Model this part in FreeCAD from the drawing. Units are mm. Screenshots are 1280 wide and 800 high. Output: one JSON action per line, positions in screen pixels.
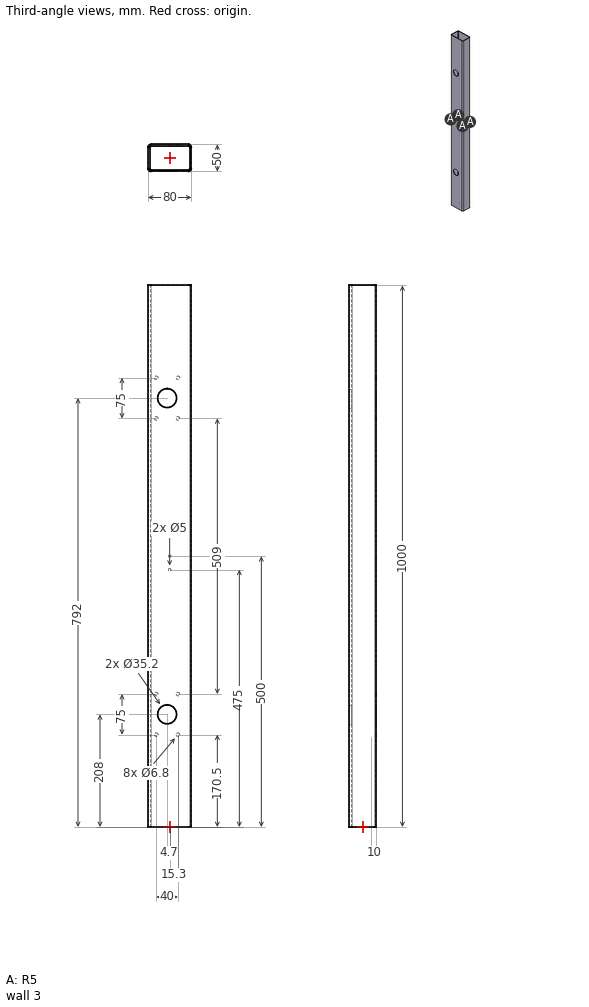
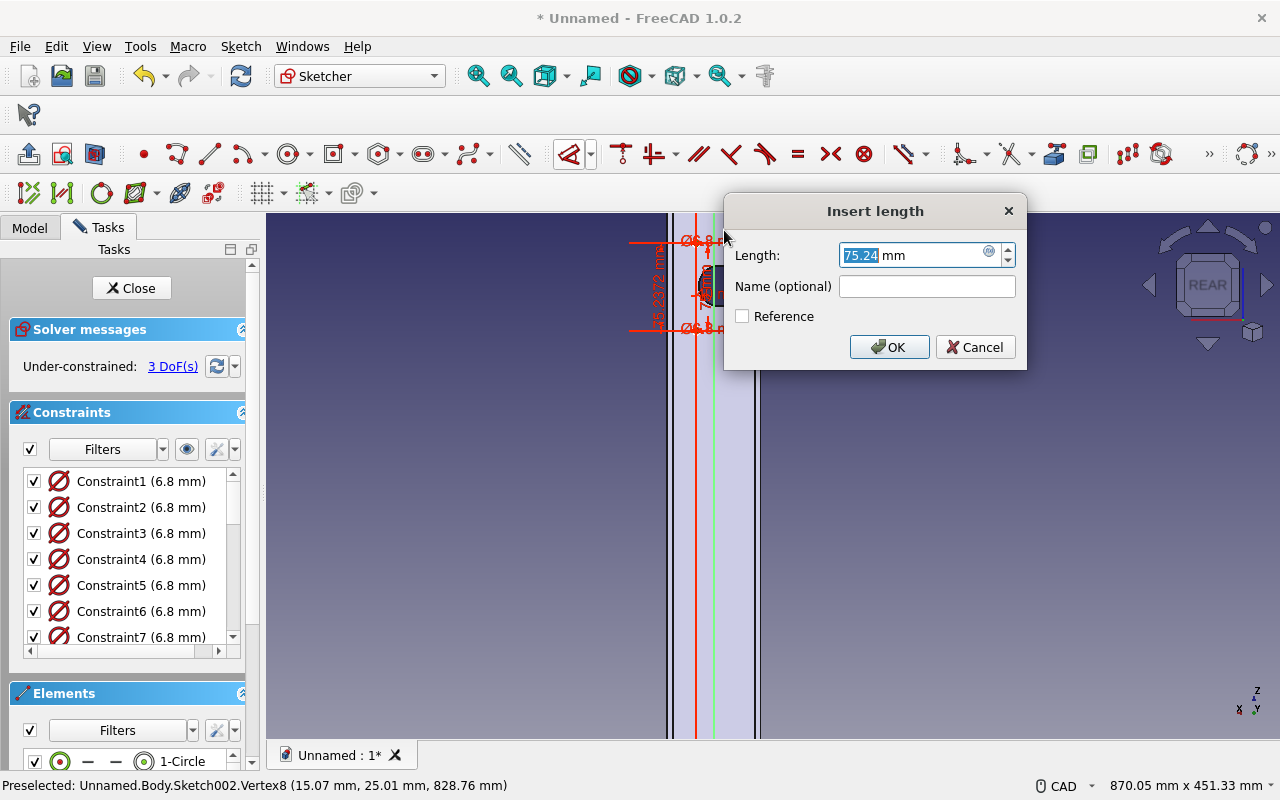
{"action": "type", "text": "75"}
{"action": "key", "text": "Return"}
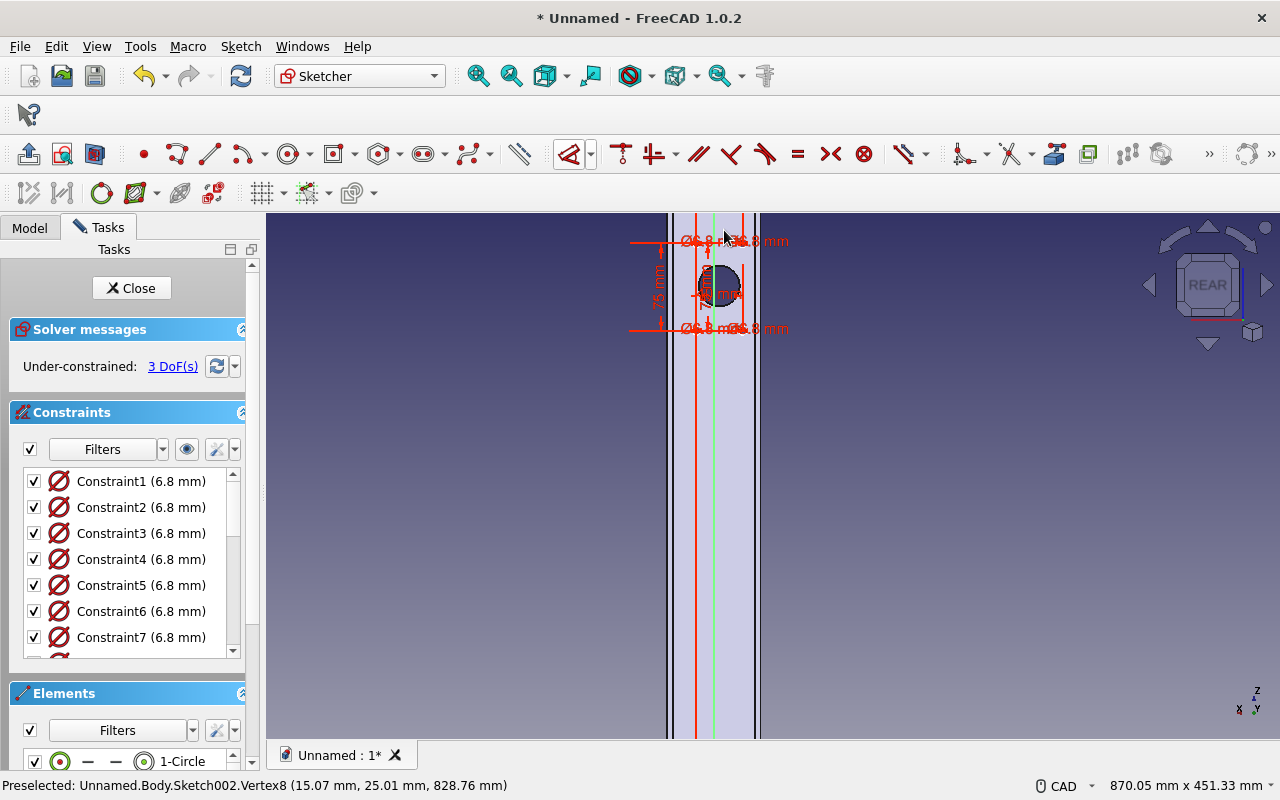
{"action": "scroll", "coordinate": [696, 332], "scroll_direction": "down", "scroll_amount": 5}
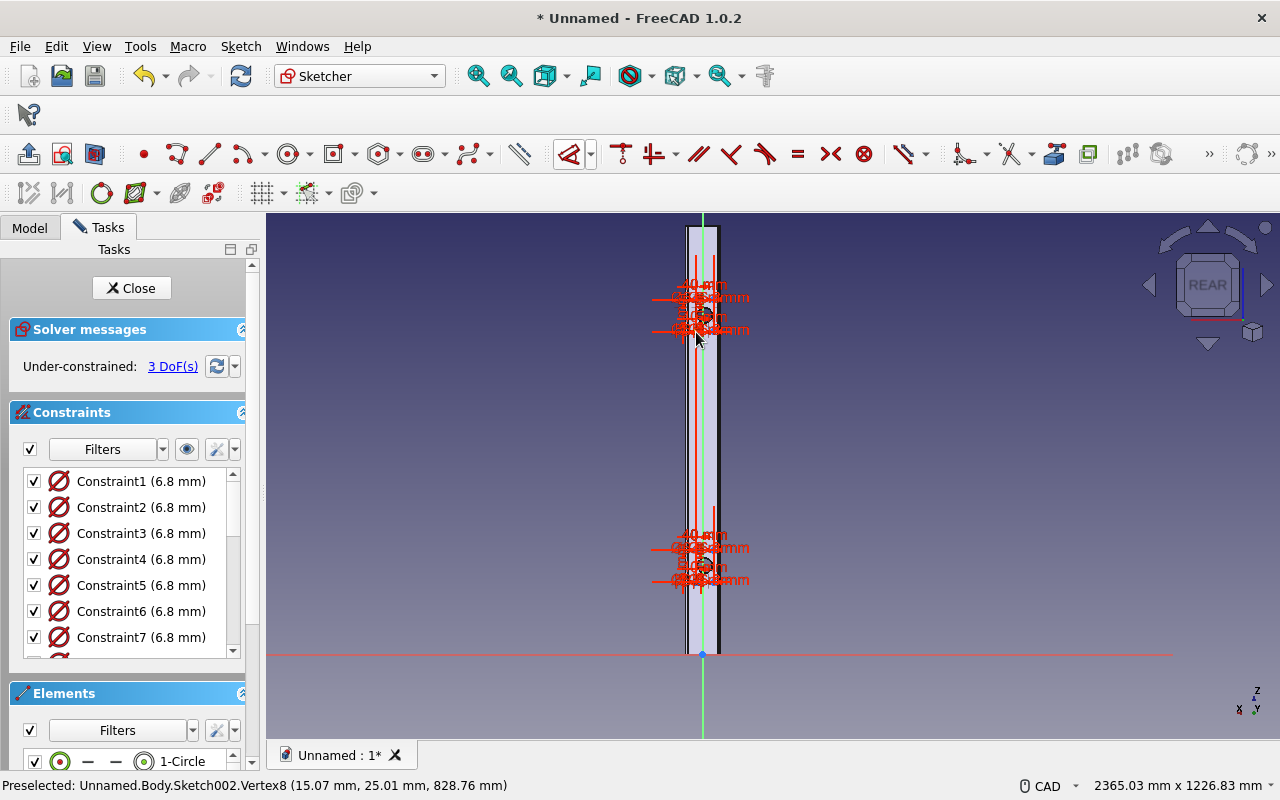
{"action": "scroll", "coordinate": [696, 582], "scroll_direction": "up", "scroll_amount": 10}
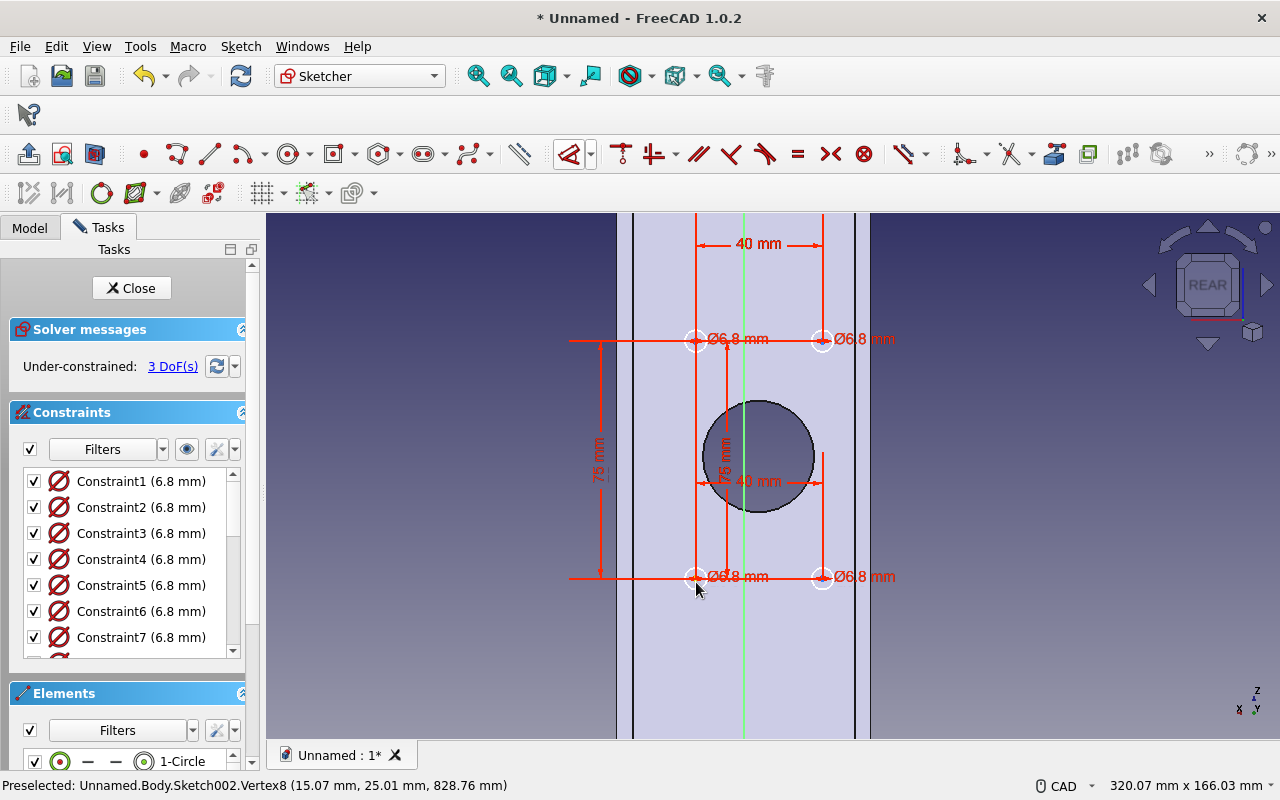
{"action": "left_click", "coordinate": [696, 579]}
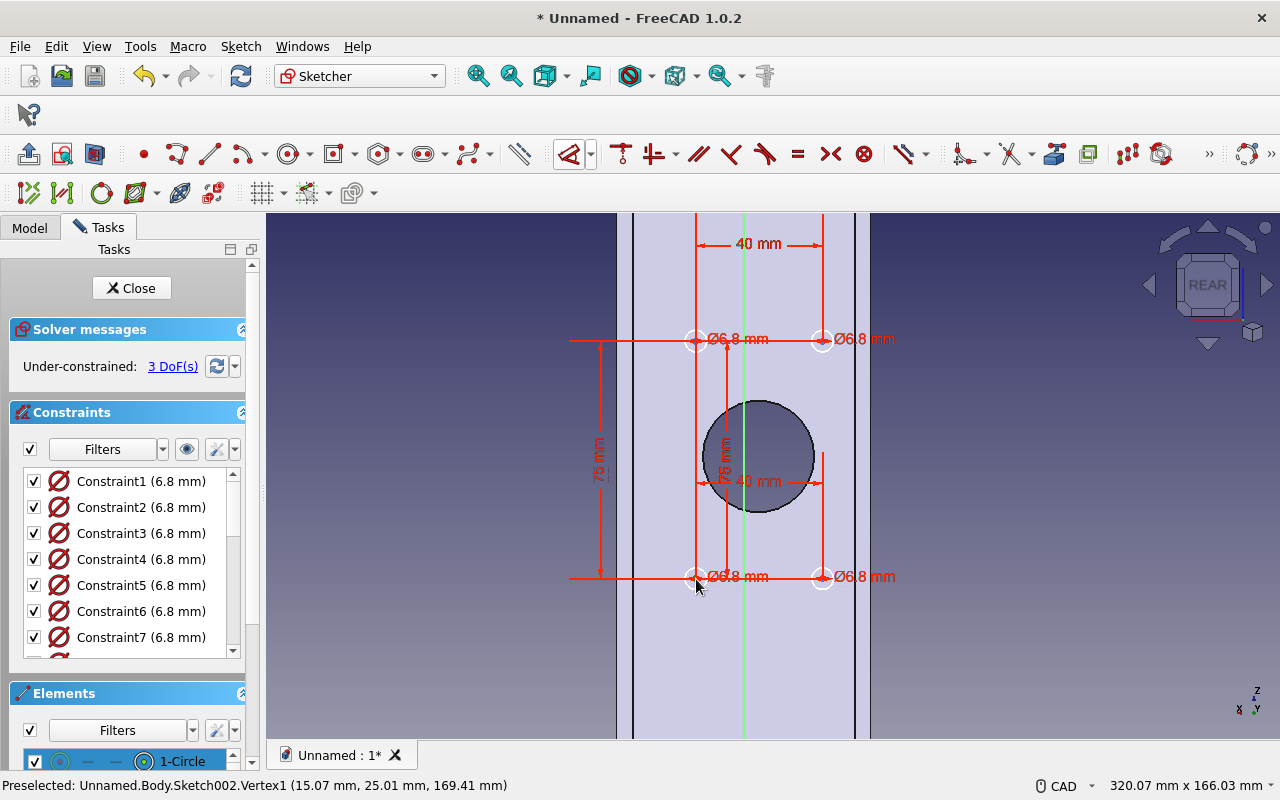
{"action": "left_click", "coordinate": [590, 154]}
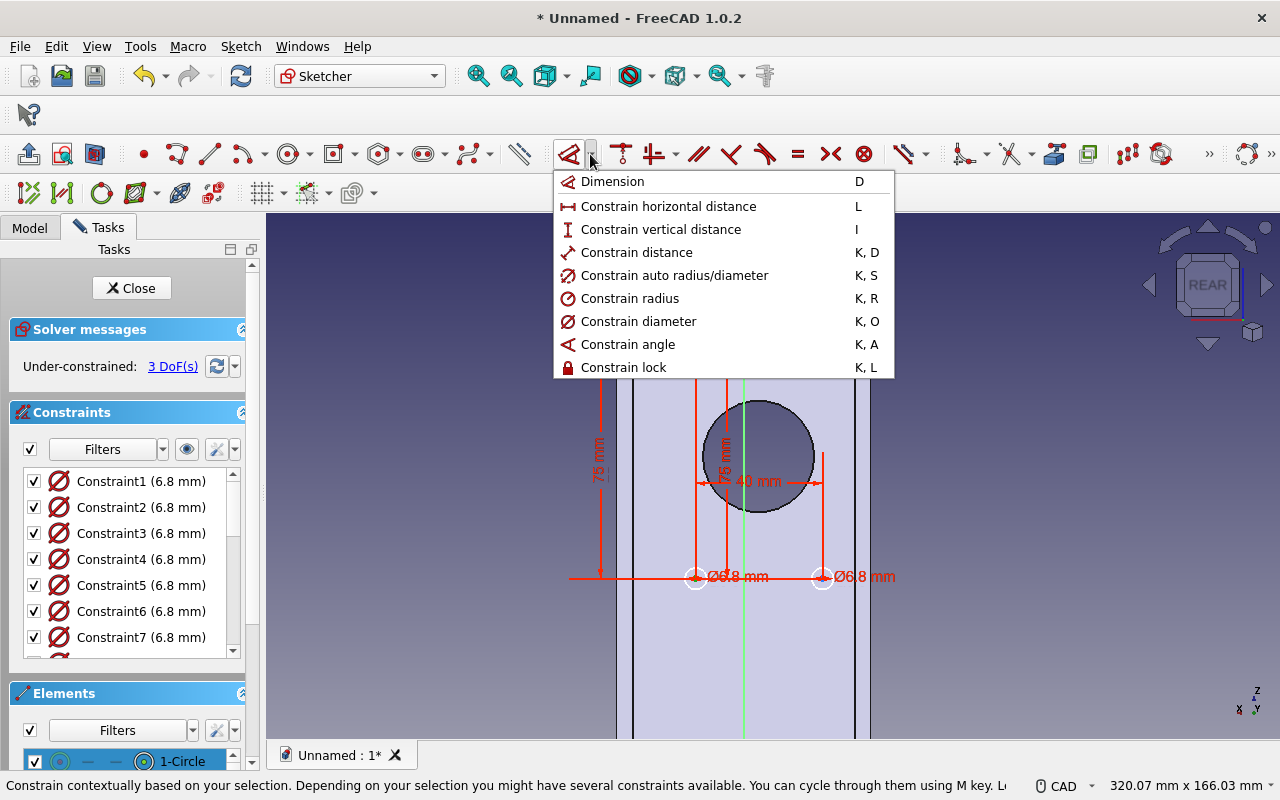
{"action": "left_click", "coordinate": [724, 206]}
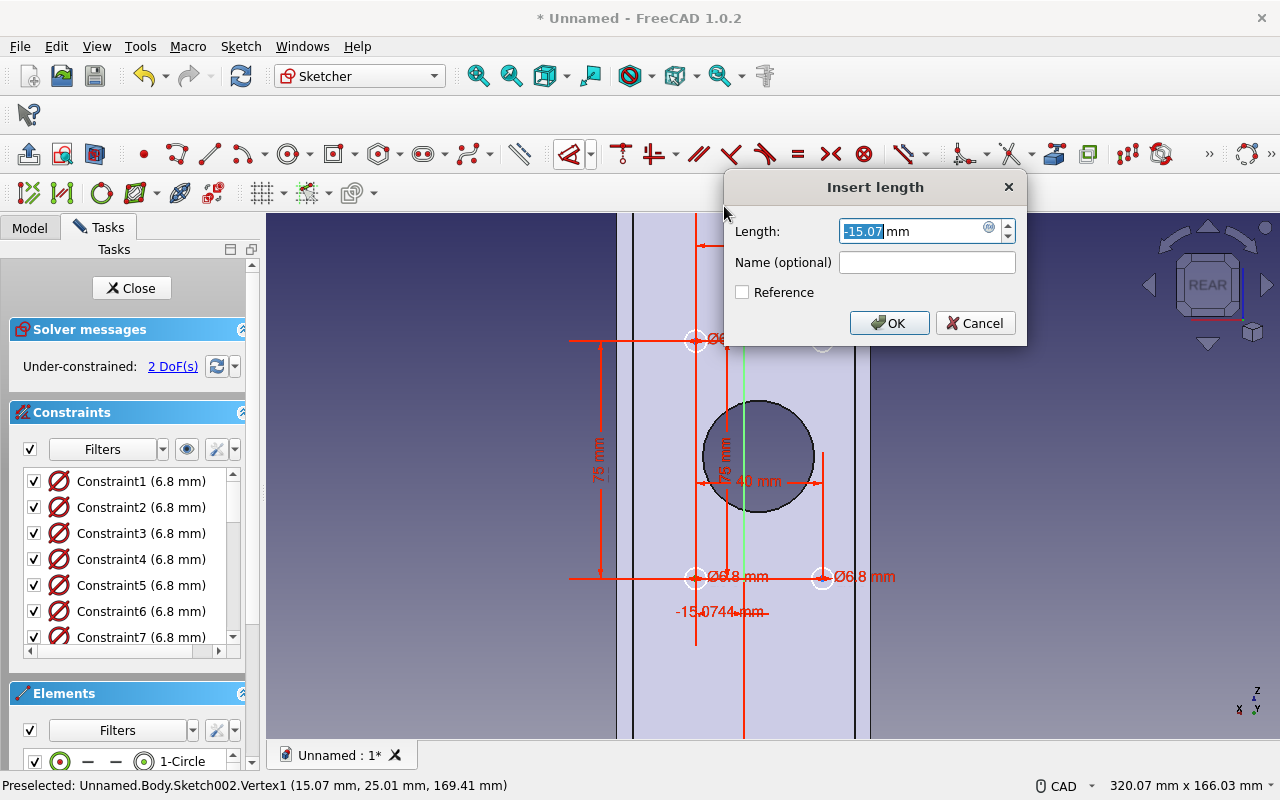
{"action": "type", "text": "-15.3"}
{"action": "key", "text": "Return"}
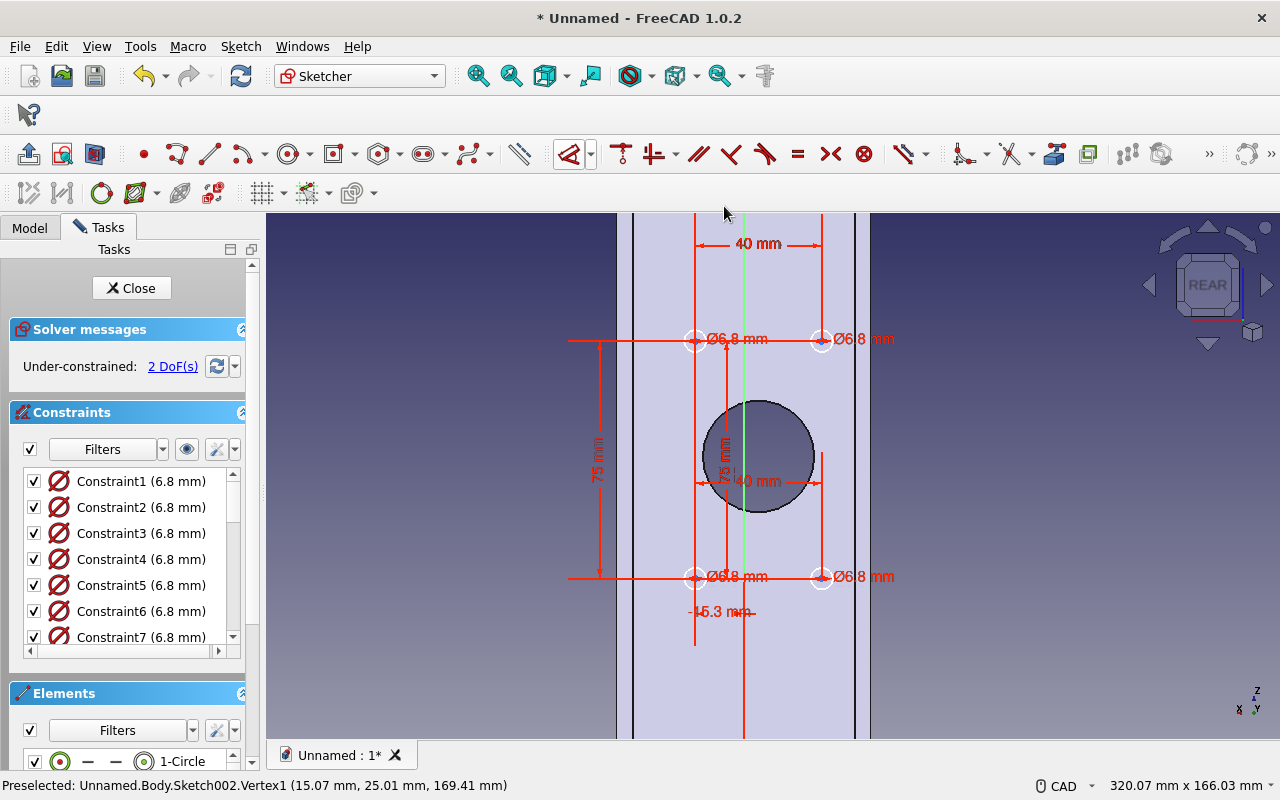
{"action": "scroll", "coordinate": [696, 582], "scroll_direction": "down", "scroll_amount": 10}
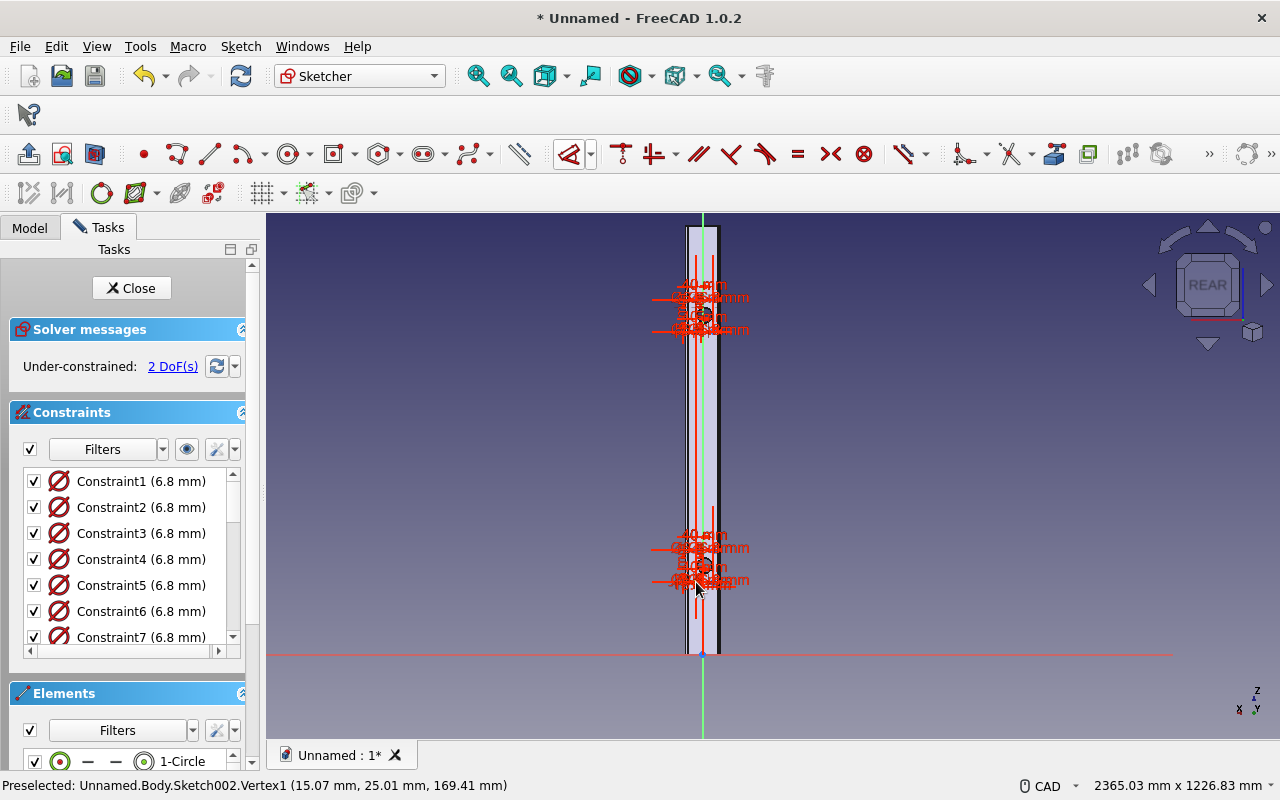
{"action": "left_click", "coordinate": [696, 550]}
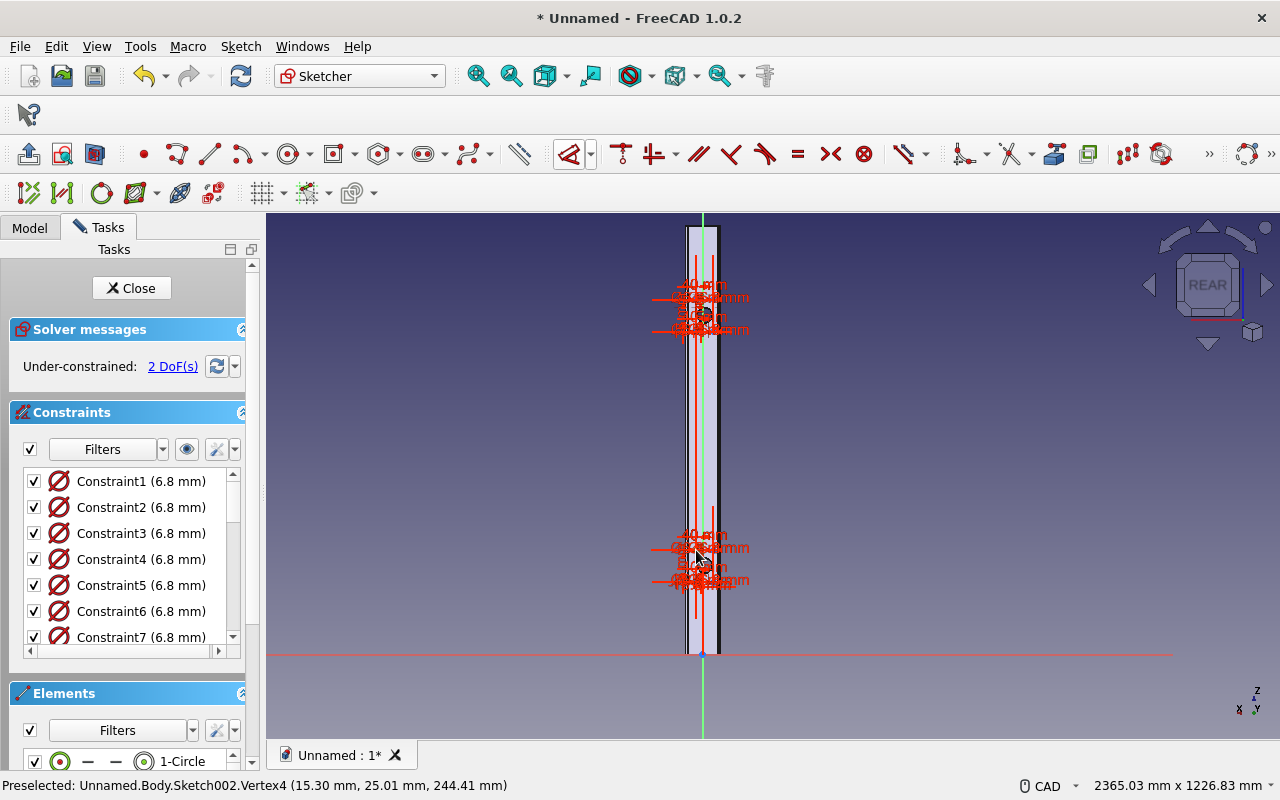
{"action": "left_click", "coordinate": [696, 332]}